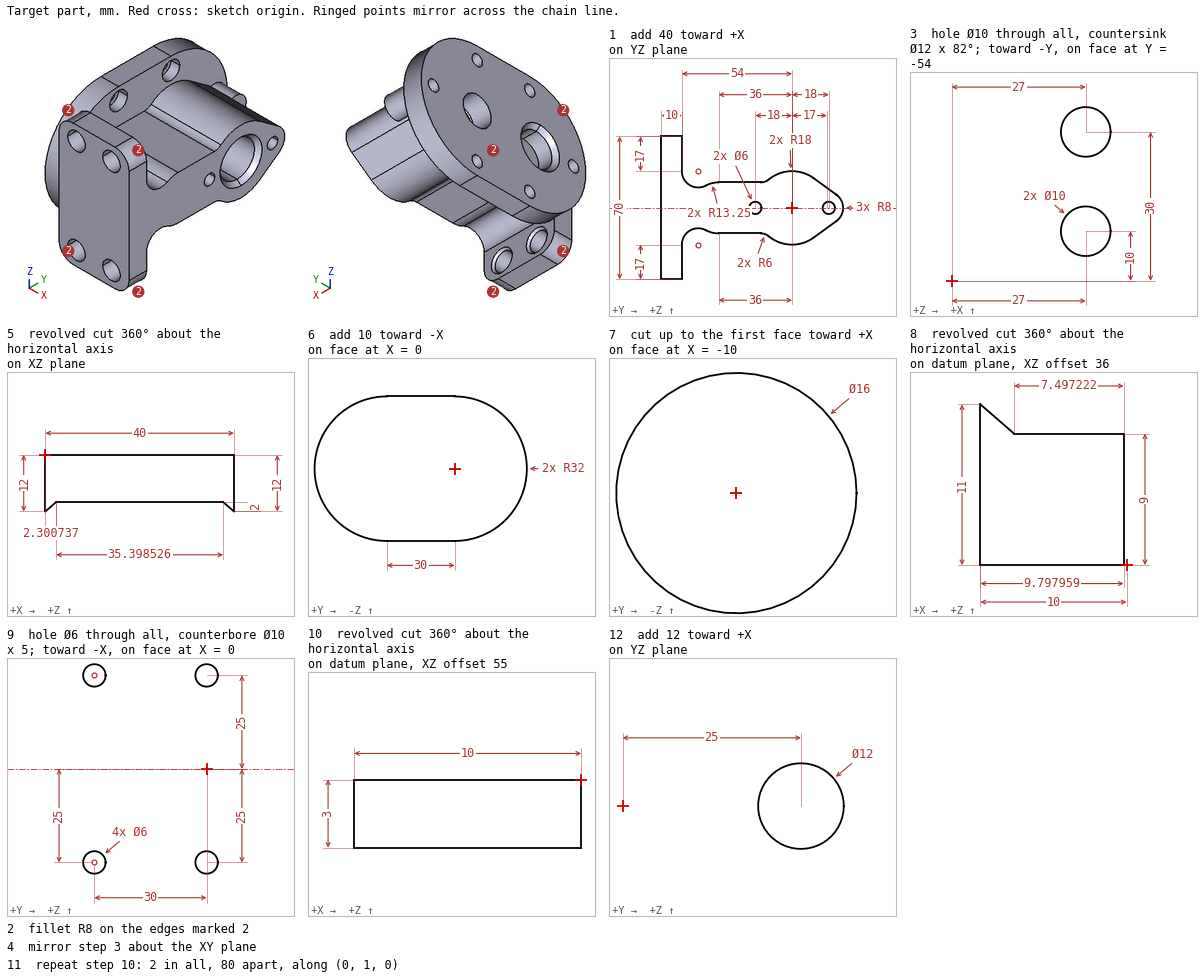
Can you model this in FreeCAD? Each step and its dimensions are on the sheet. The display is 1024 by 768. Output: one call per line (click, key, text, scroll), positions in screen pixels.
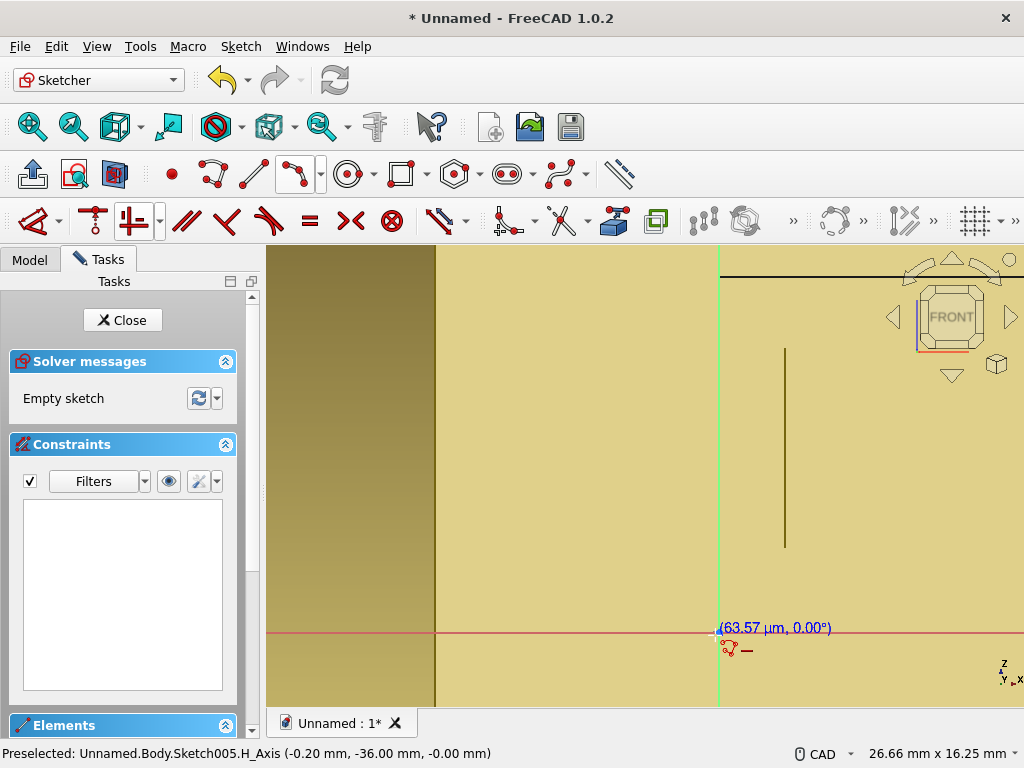
click(435, 624)
click(435, 320)
click(500, 377)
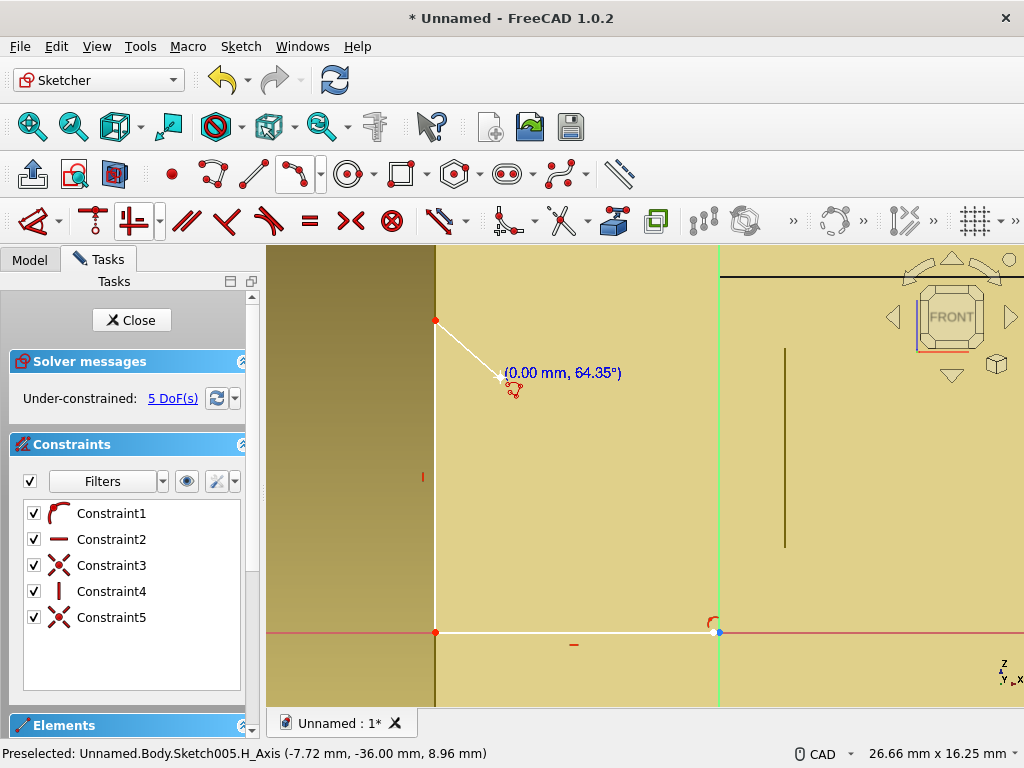
scroll(714, 377, up, 6)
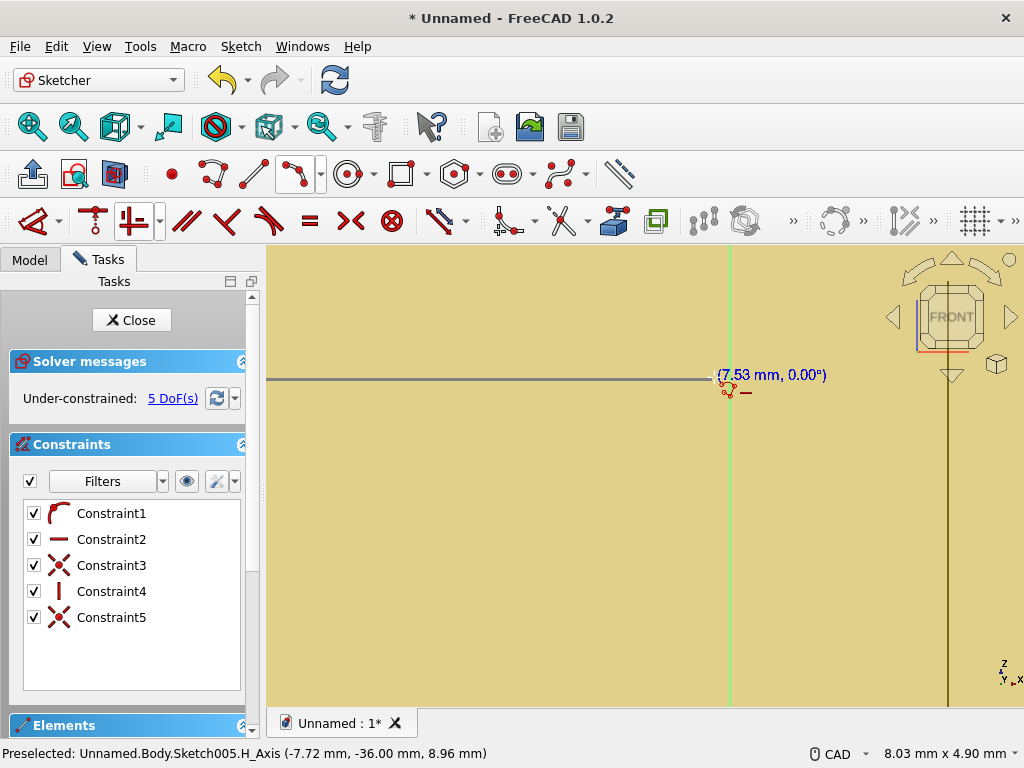
click(711, 376)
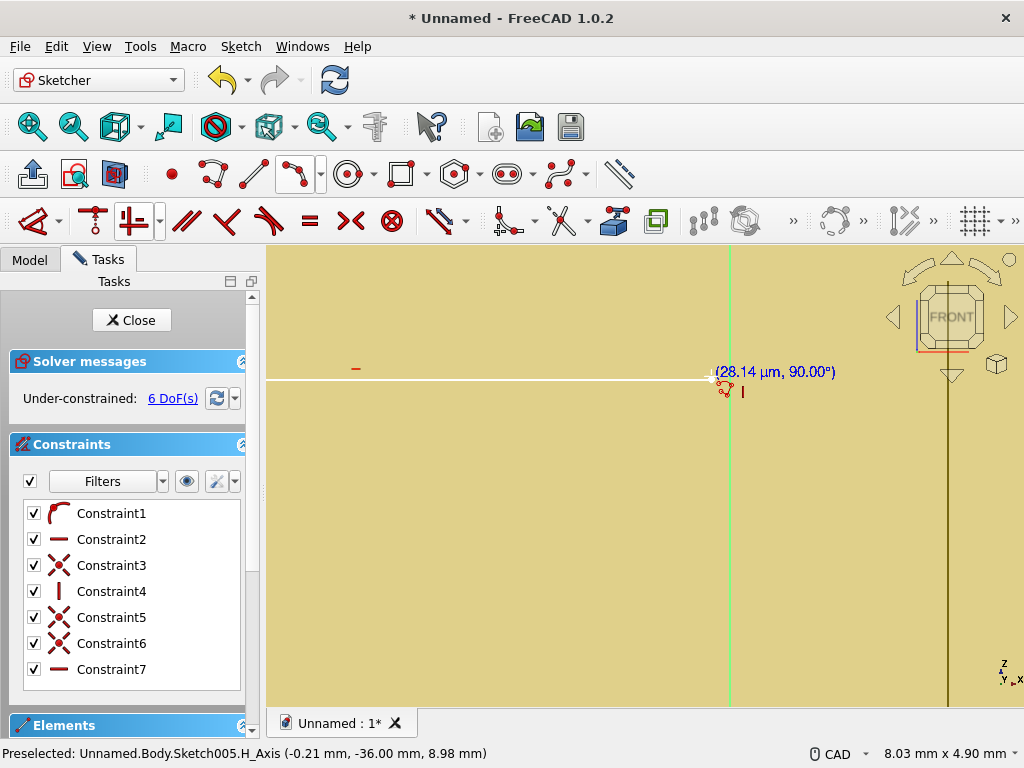
scroll(714, 377, down, 6)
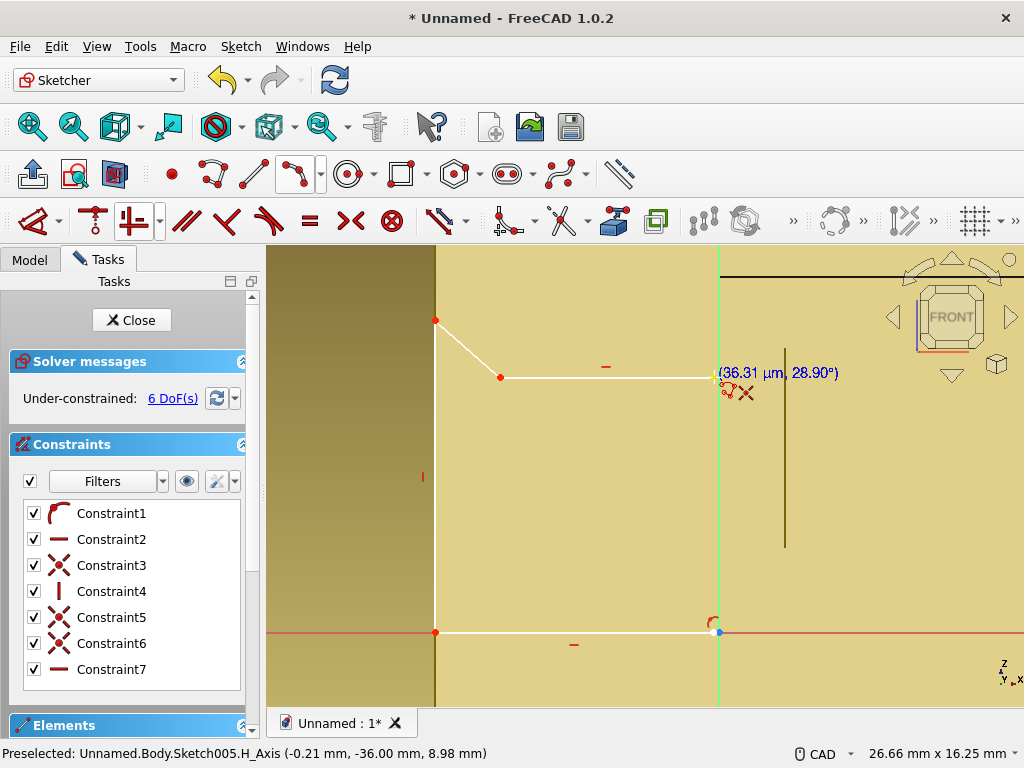
scroll(714, 633, up, 6)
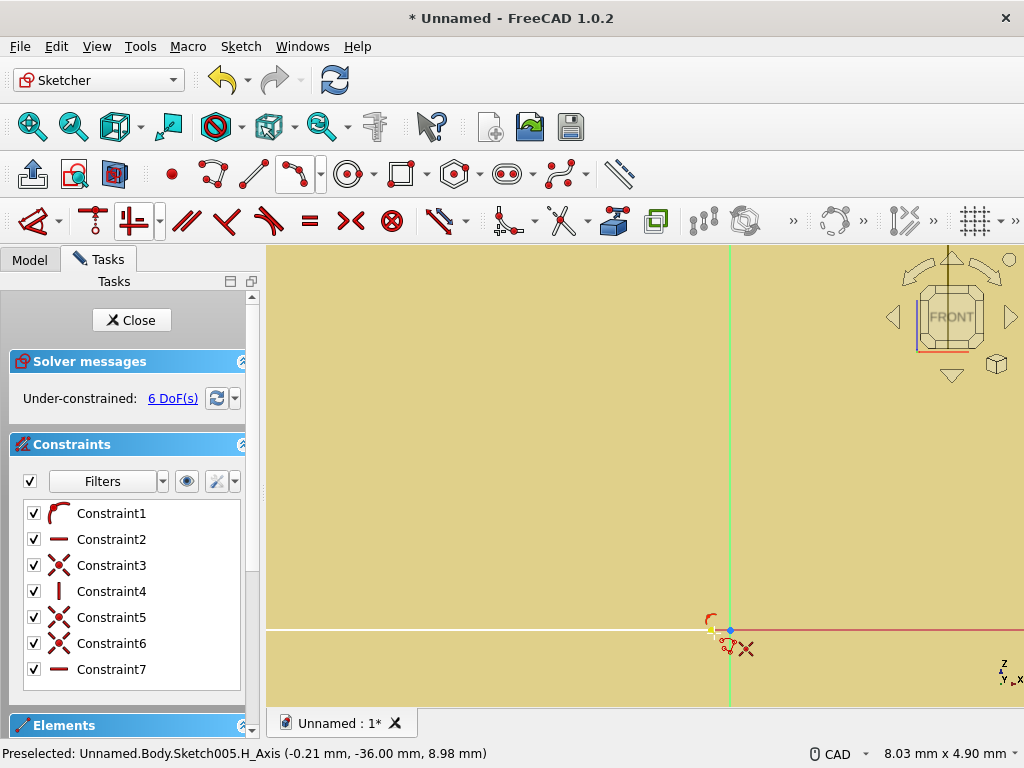
click(711, 630)
key(Escape)
key(Escape)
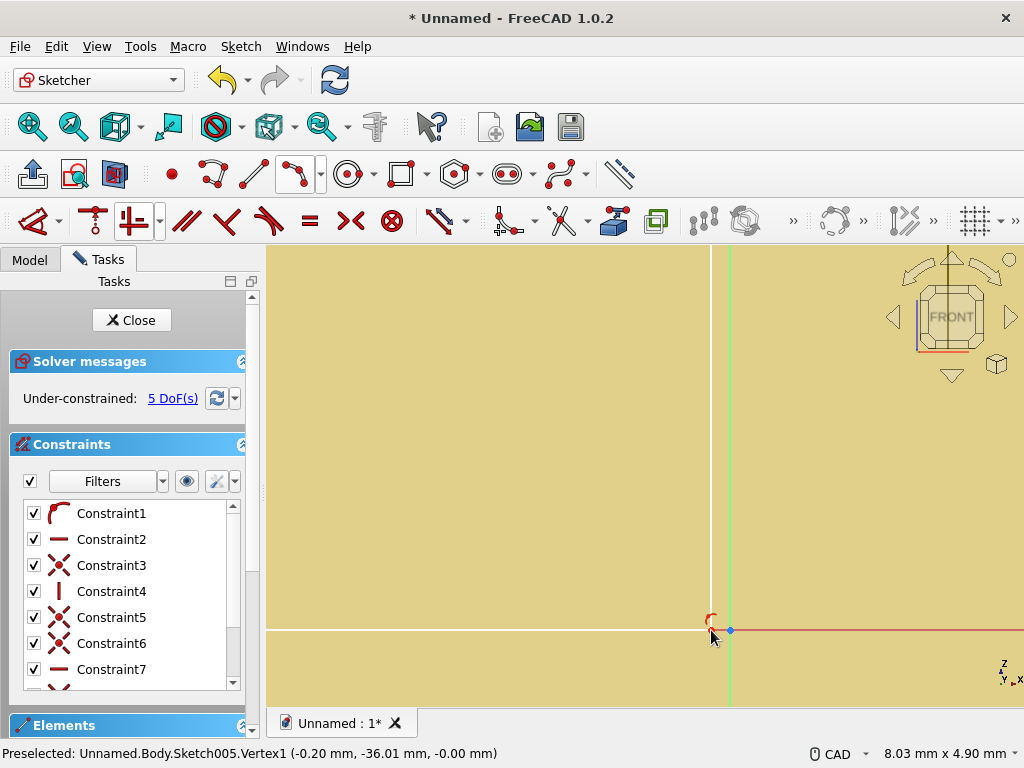
click(32, 222)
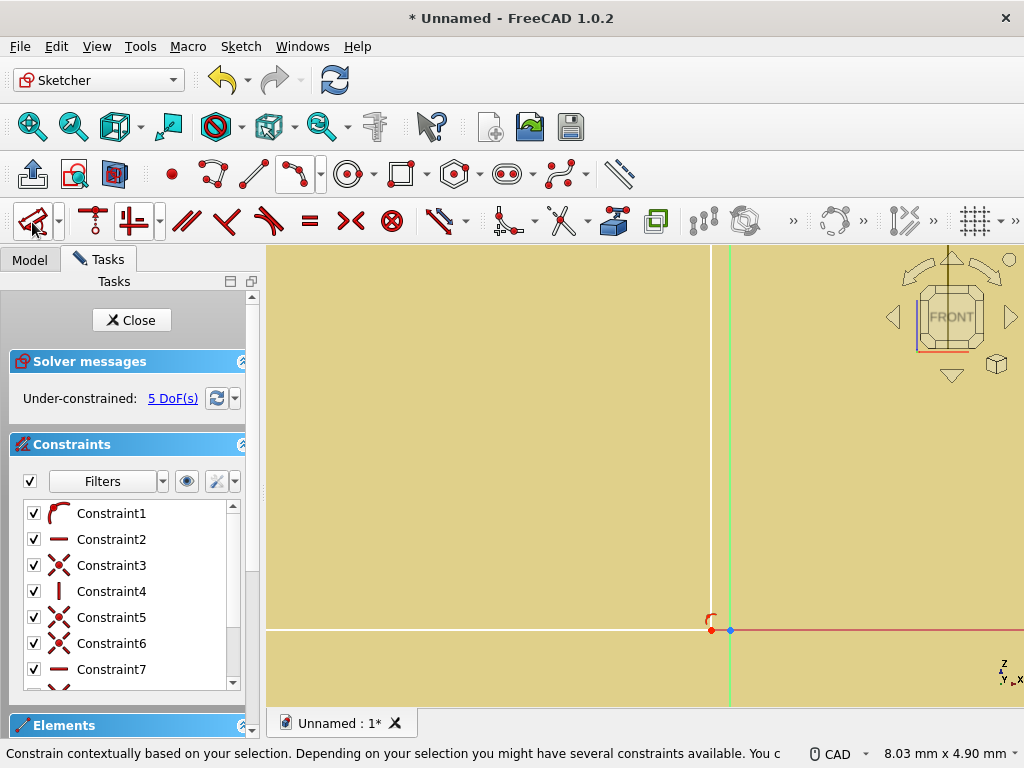
click(711, 377)
click(745, 452)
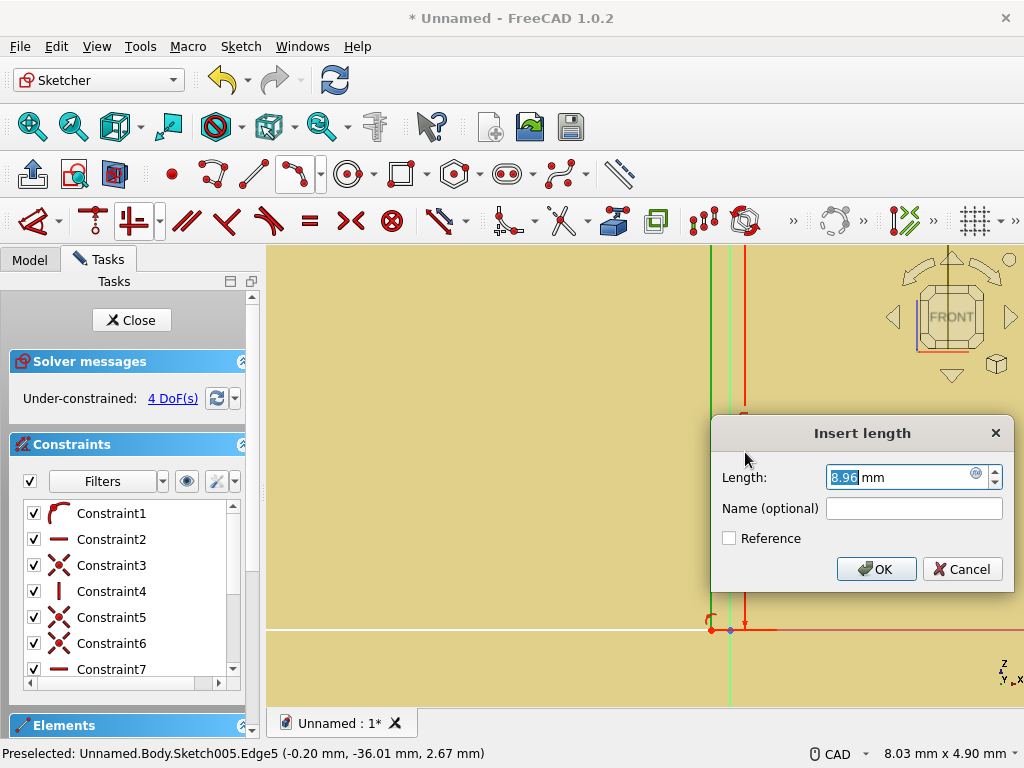
text(9)
key(Return)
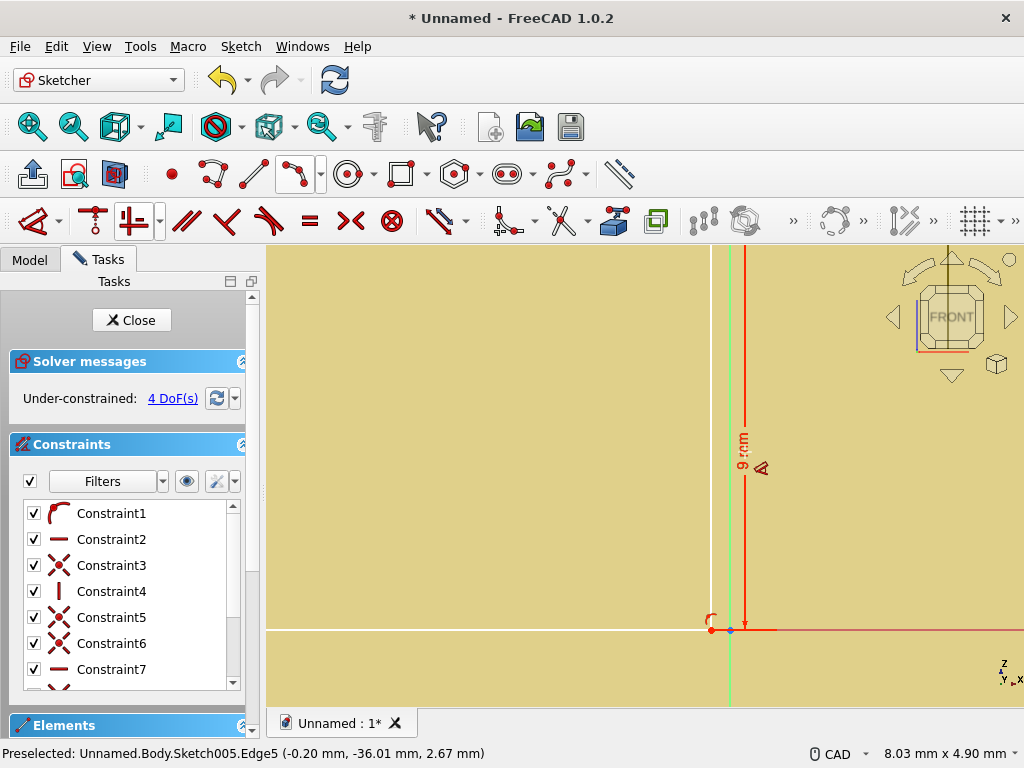
scroll(714, 633, down, 6)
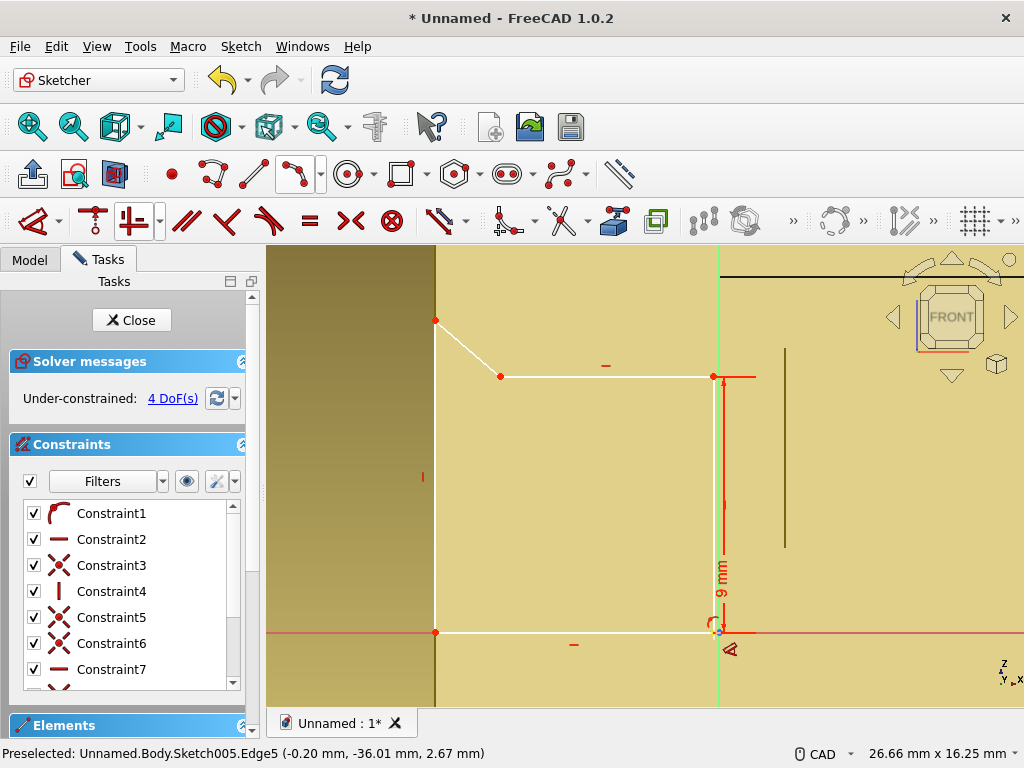
click(435, 539)
click(401, 477)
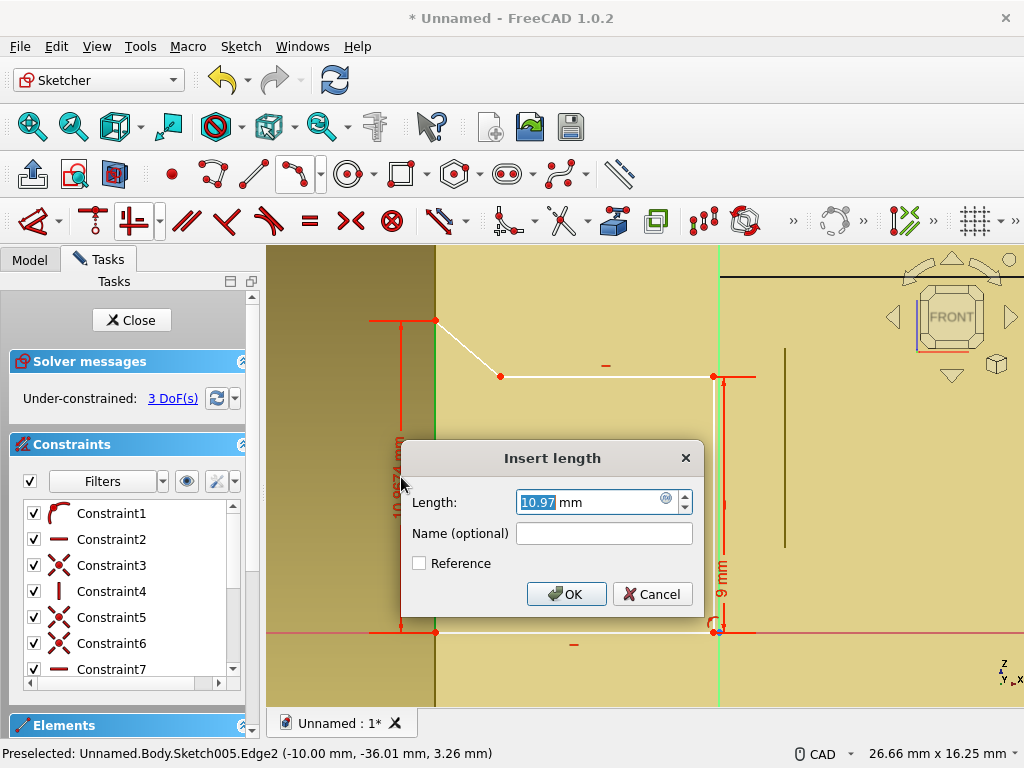
text(11)
key(Return)